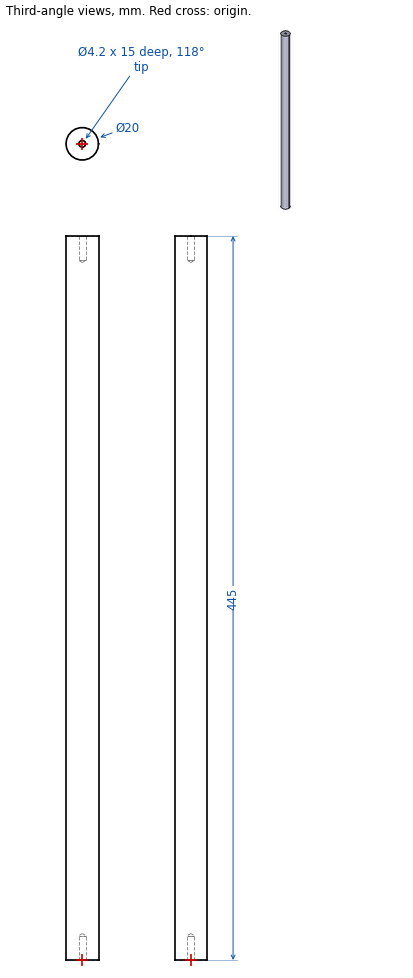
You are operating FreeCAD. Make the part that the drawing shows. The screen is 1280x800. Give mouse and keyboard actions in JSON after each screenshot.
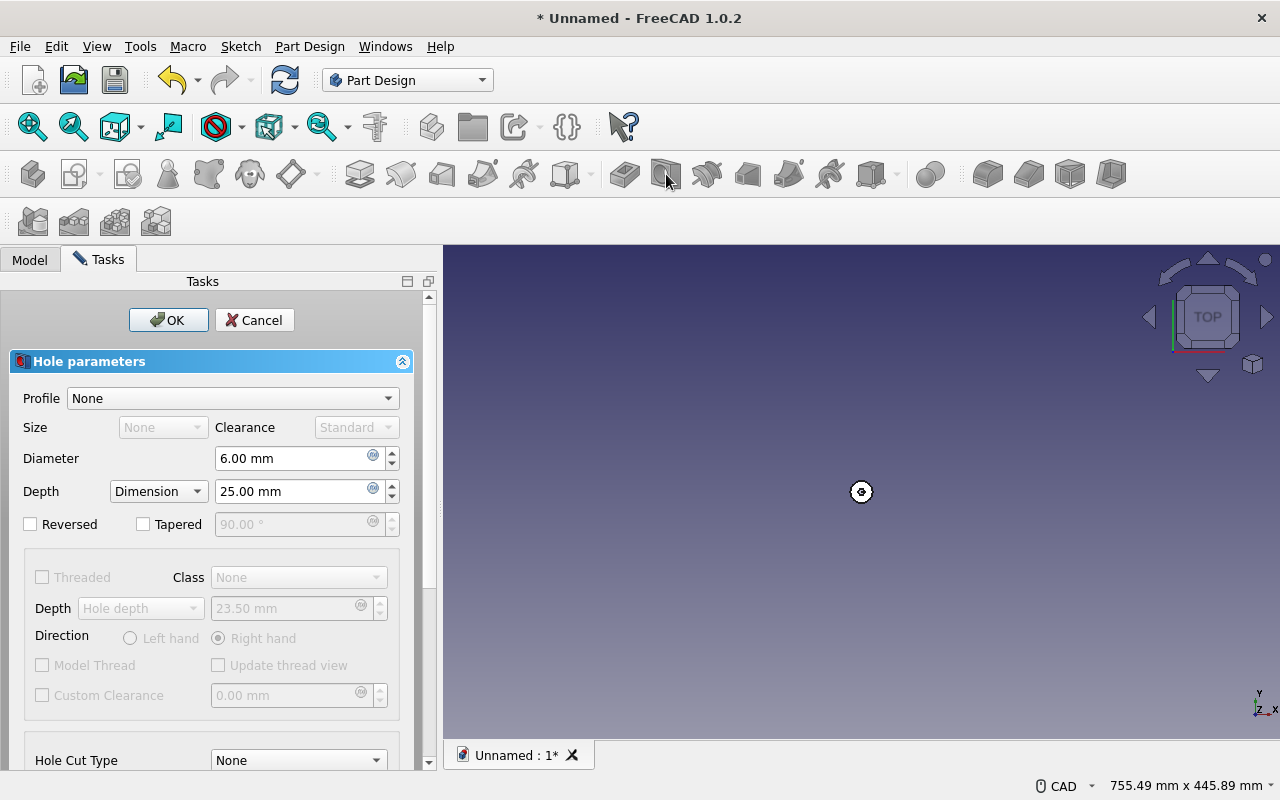
{"action": "triple_click", "coordinate": [300, 458]}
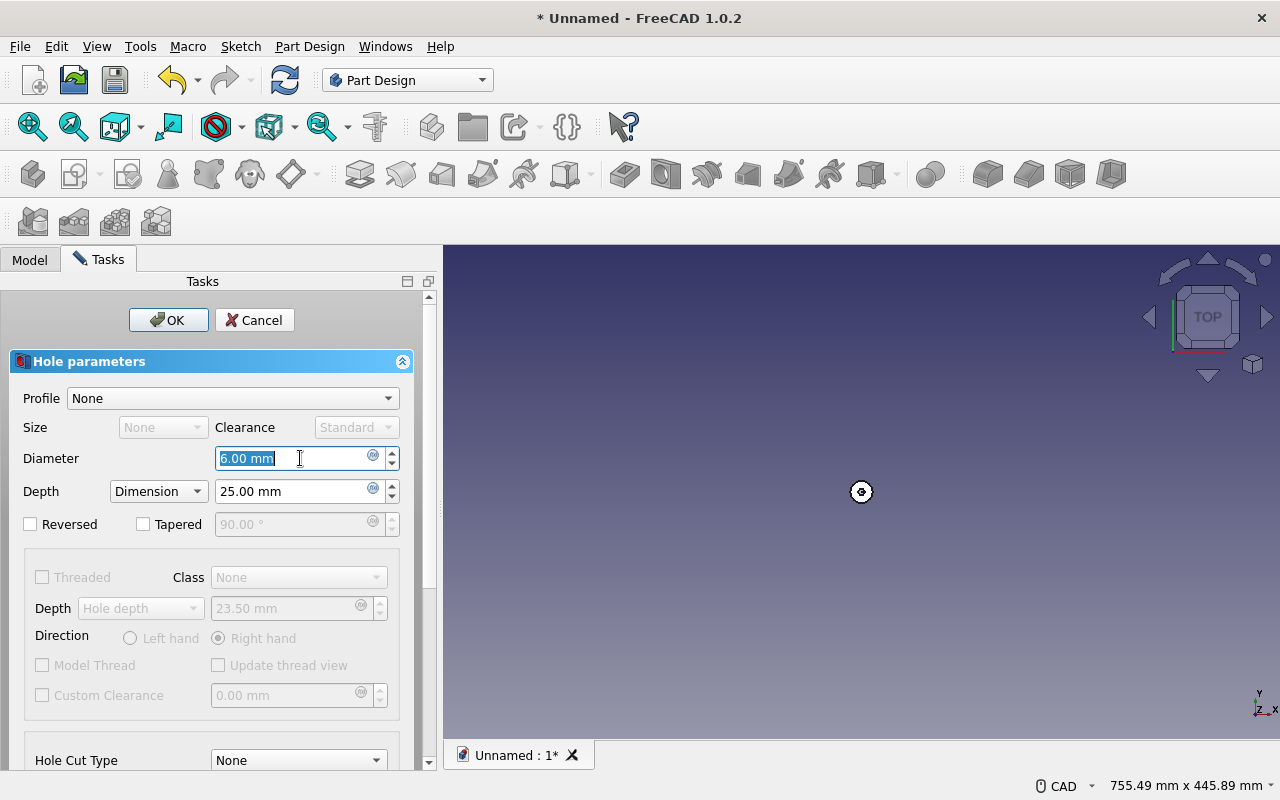
{"action": "type", "text": "4.2"}
{"action": "key", "text": "Tab"}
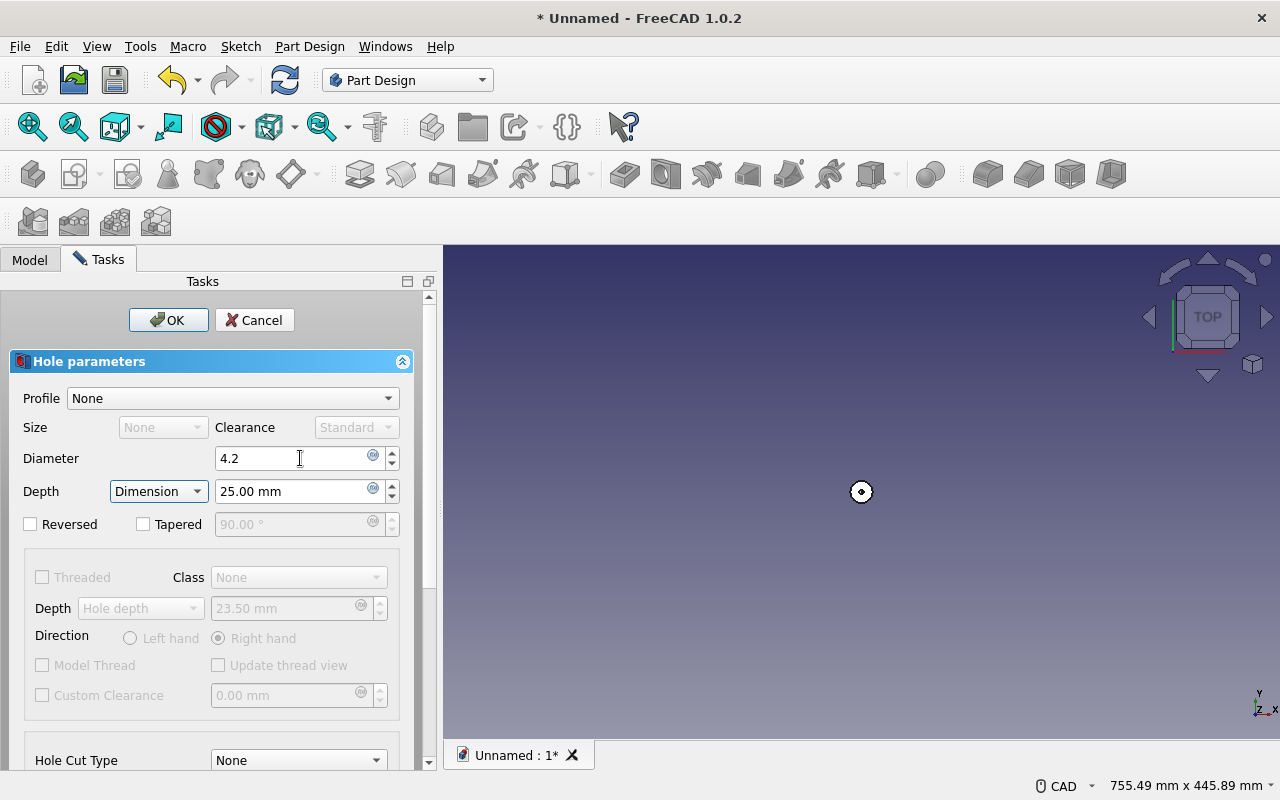
{"action": "triple_click", "coordinate": [300, 492]}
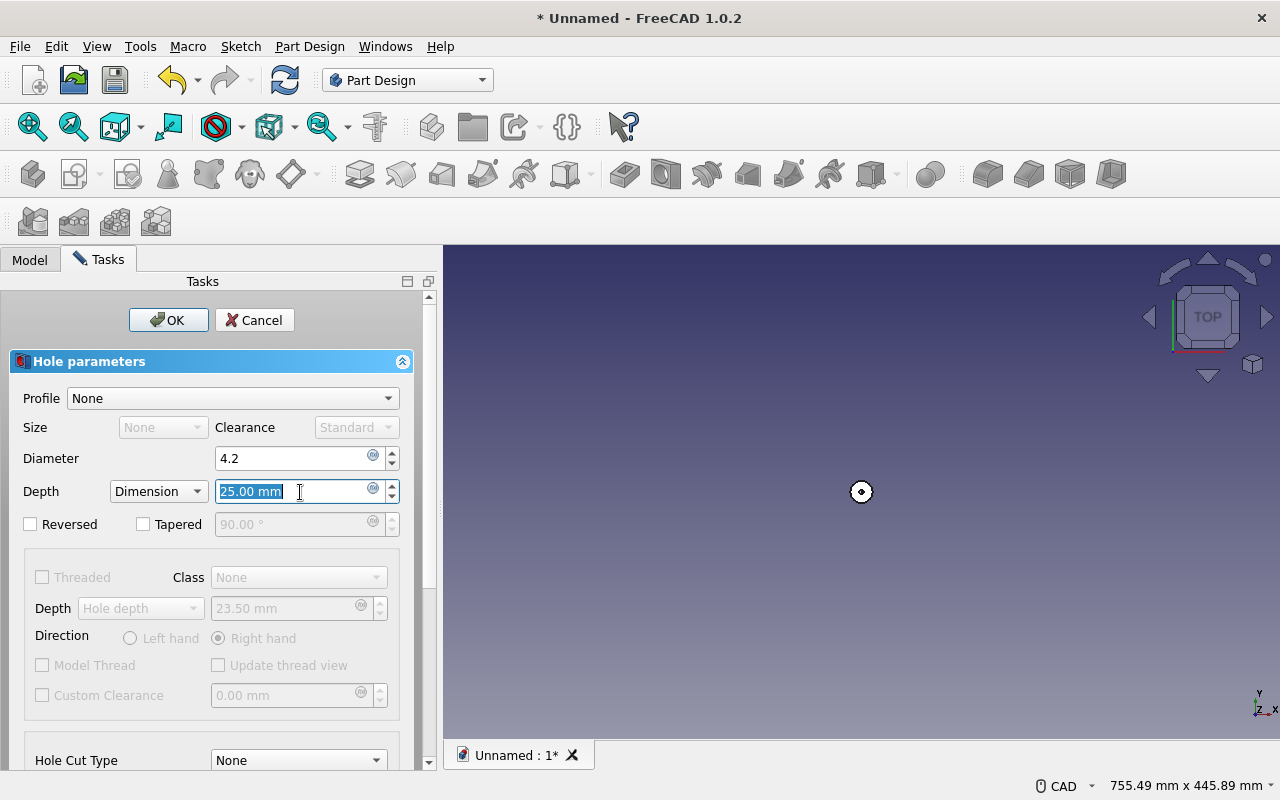
{"action": "type", "text": "15"}
{"action": "key", "text": "Tab"}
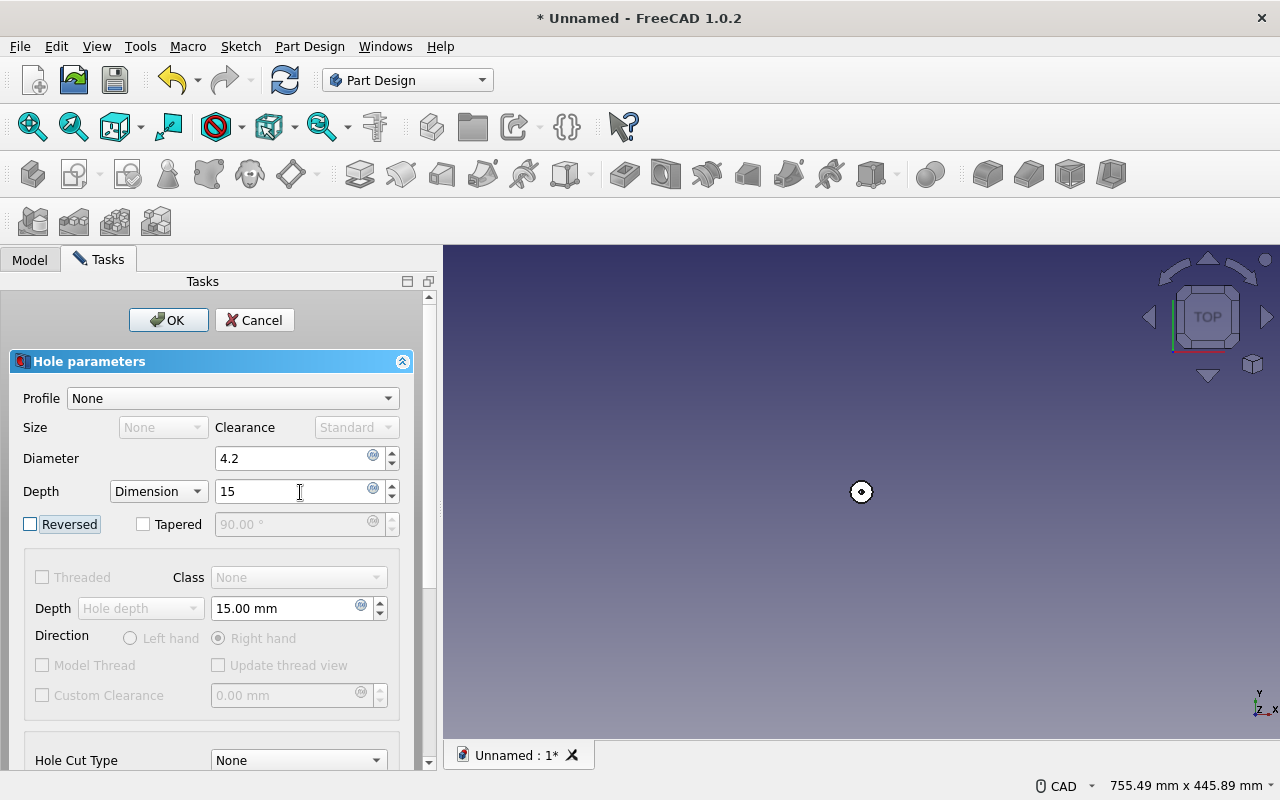
{"action": "left_click", "coordinate": [169, 320]}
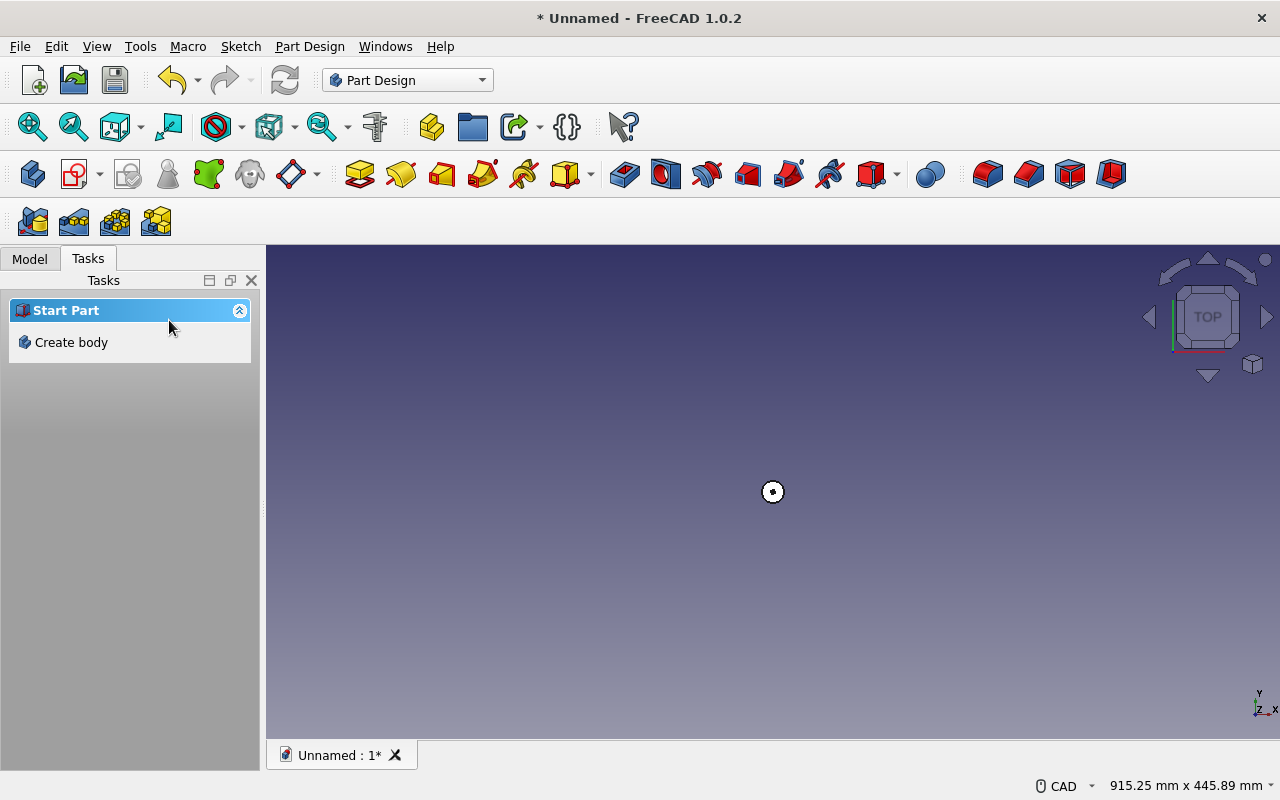
{"action": "left_click", "coordinate": [33, 128]}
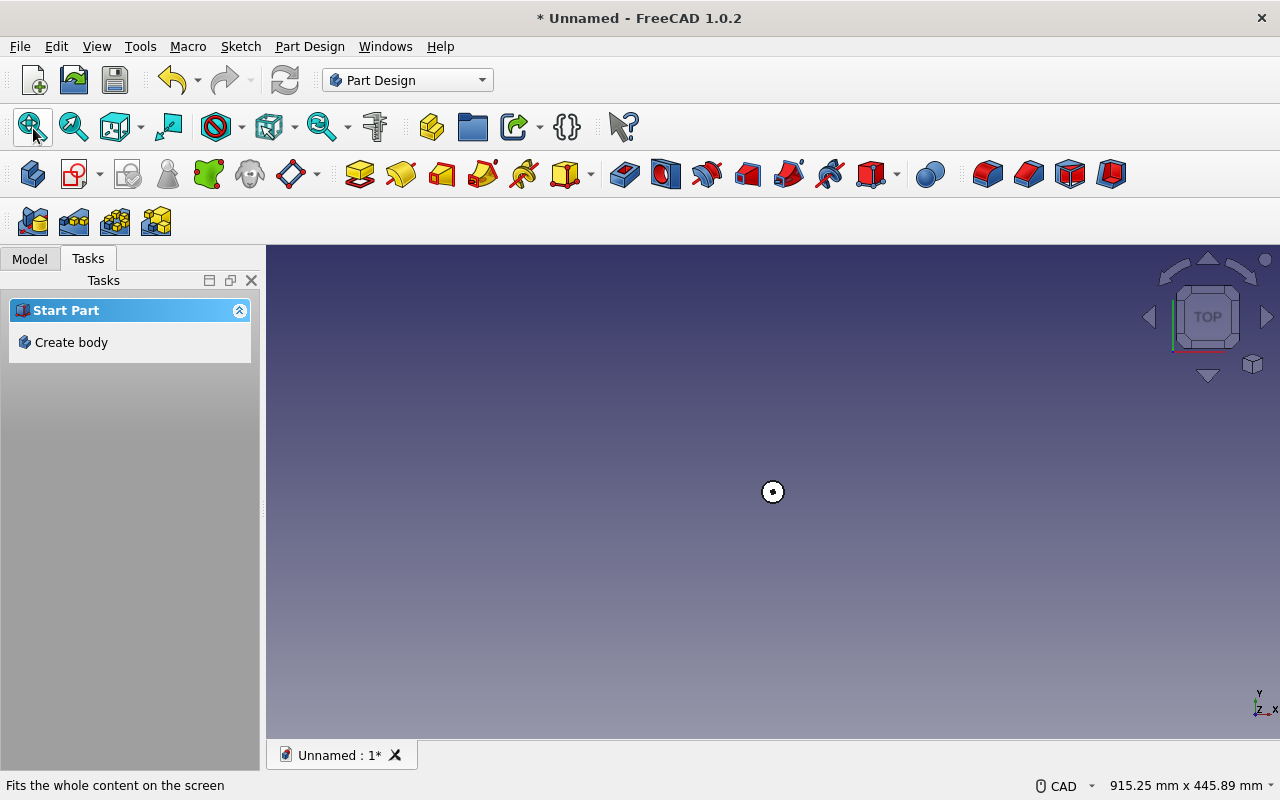
{"action": "left_click", "coordinate": [74, 174]}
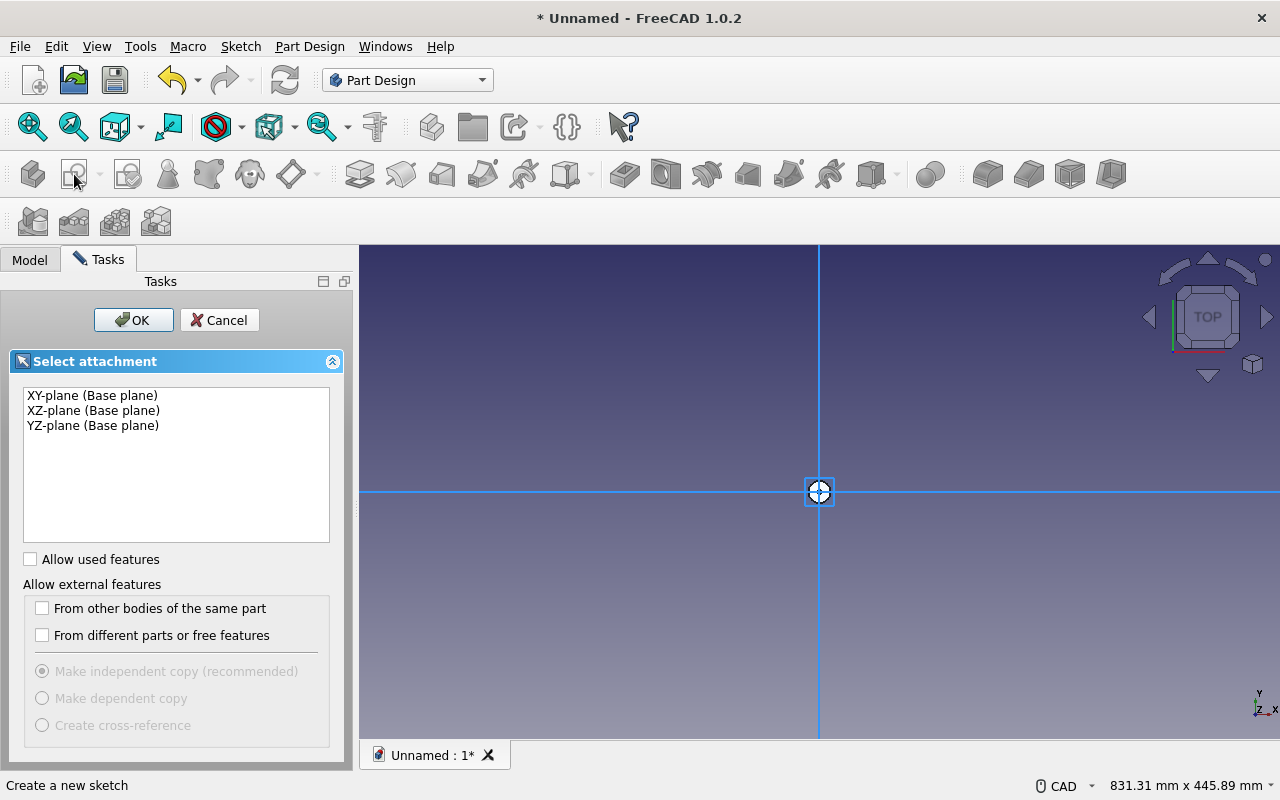
{"action": "left_click", "coordinate": [84, 396]}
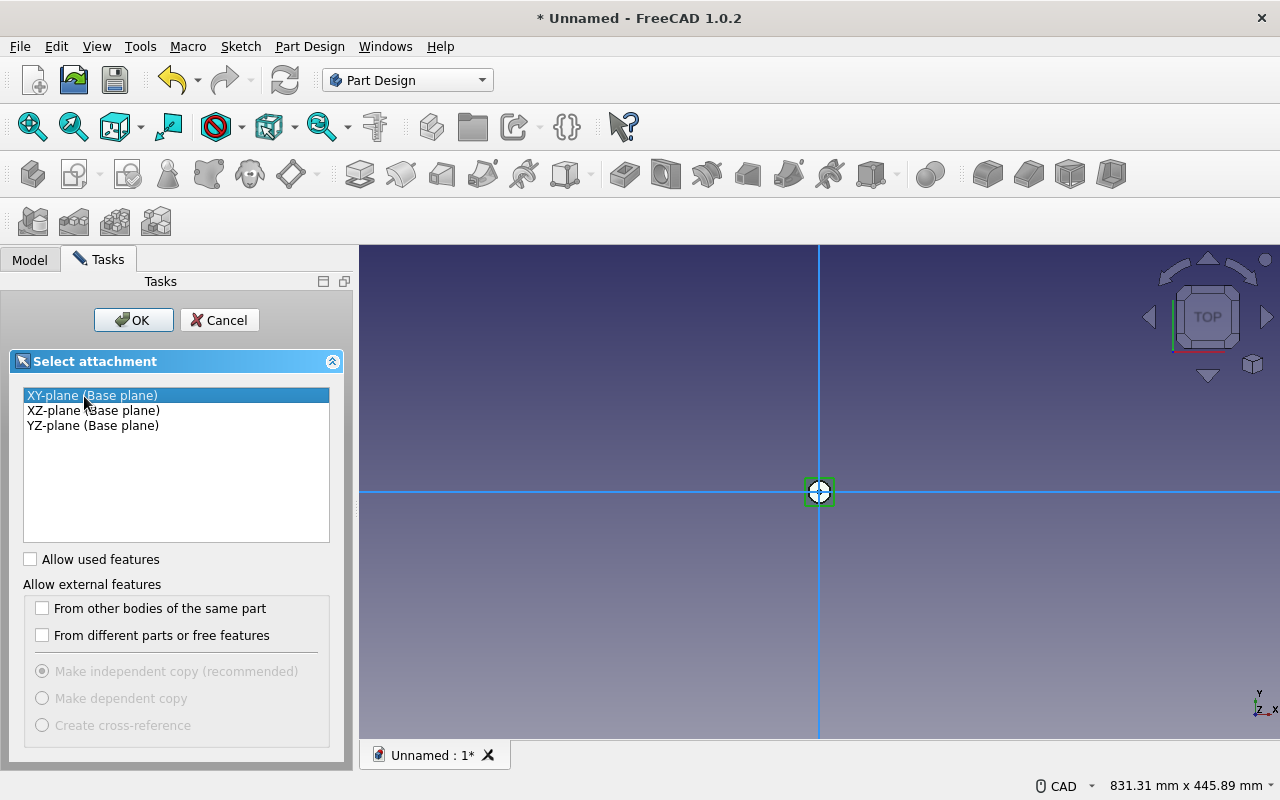
{"action": "left_click", "coordinate": [134, 320]}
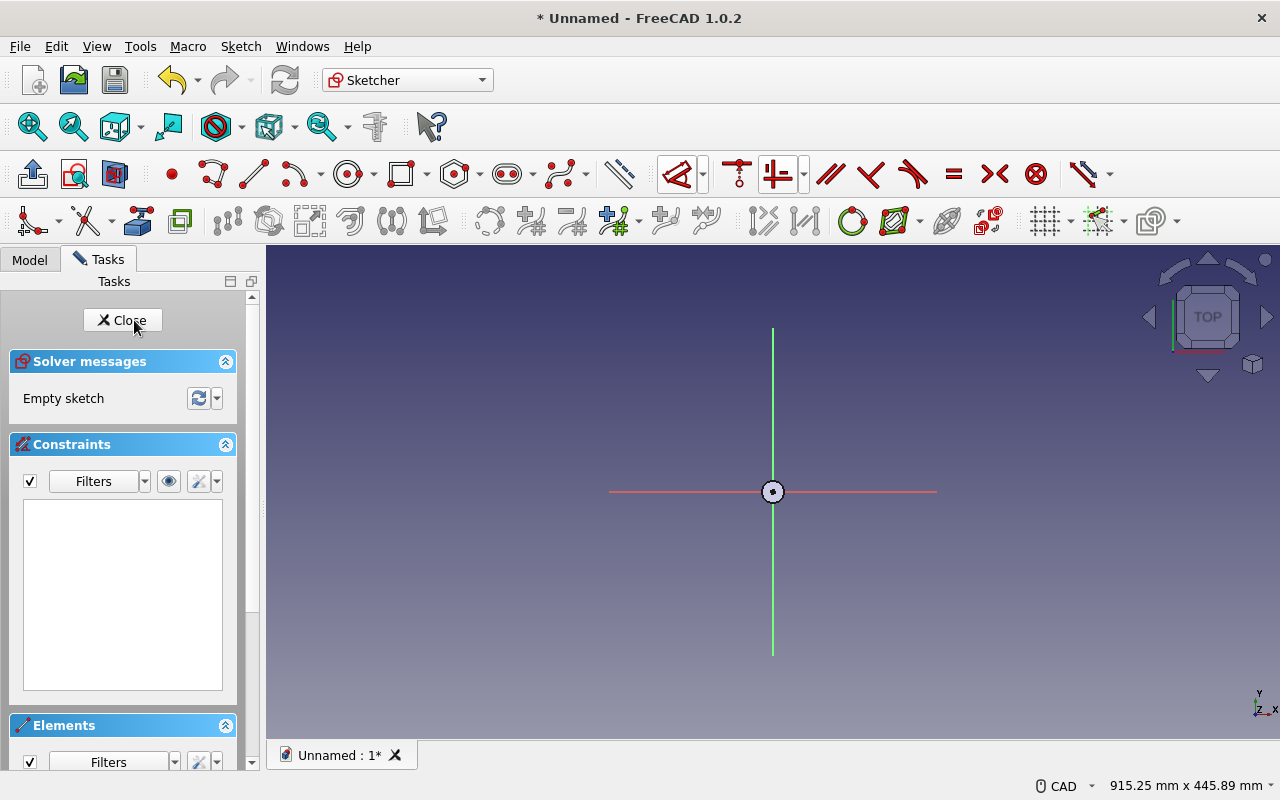
{"action": "key", "text": "q s"}